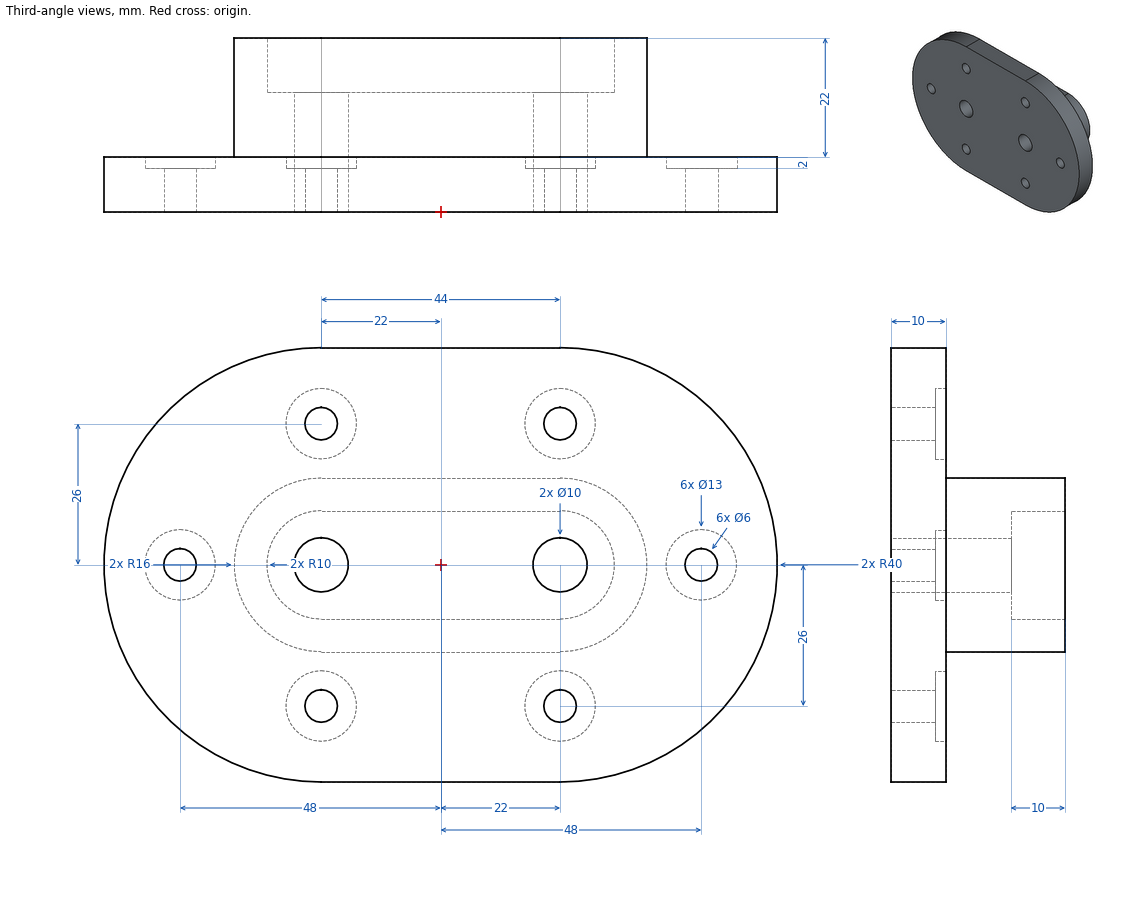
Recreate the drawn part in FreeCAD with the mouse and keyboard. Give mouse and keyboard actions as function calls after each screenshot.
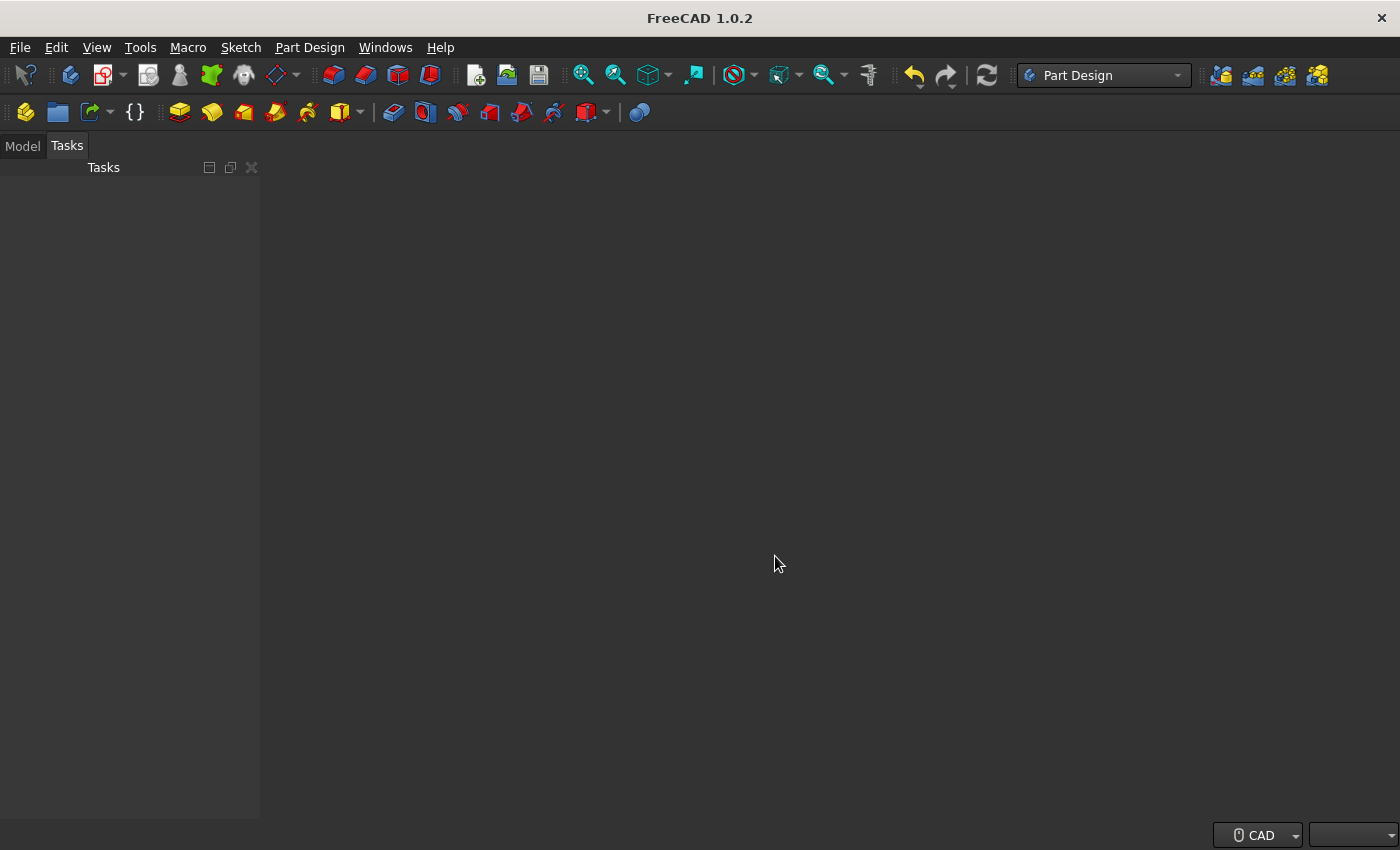
click(476, 76)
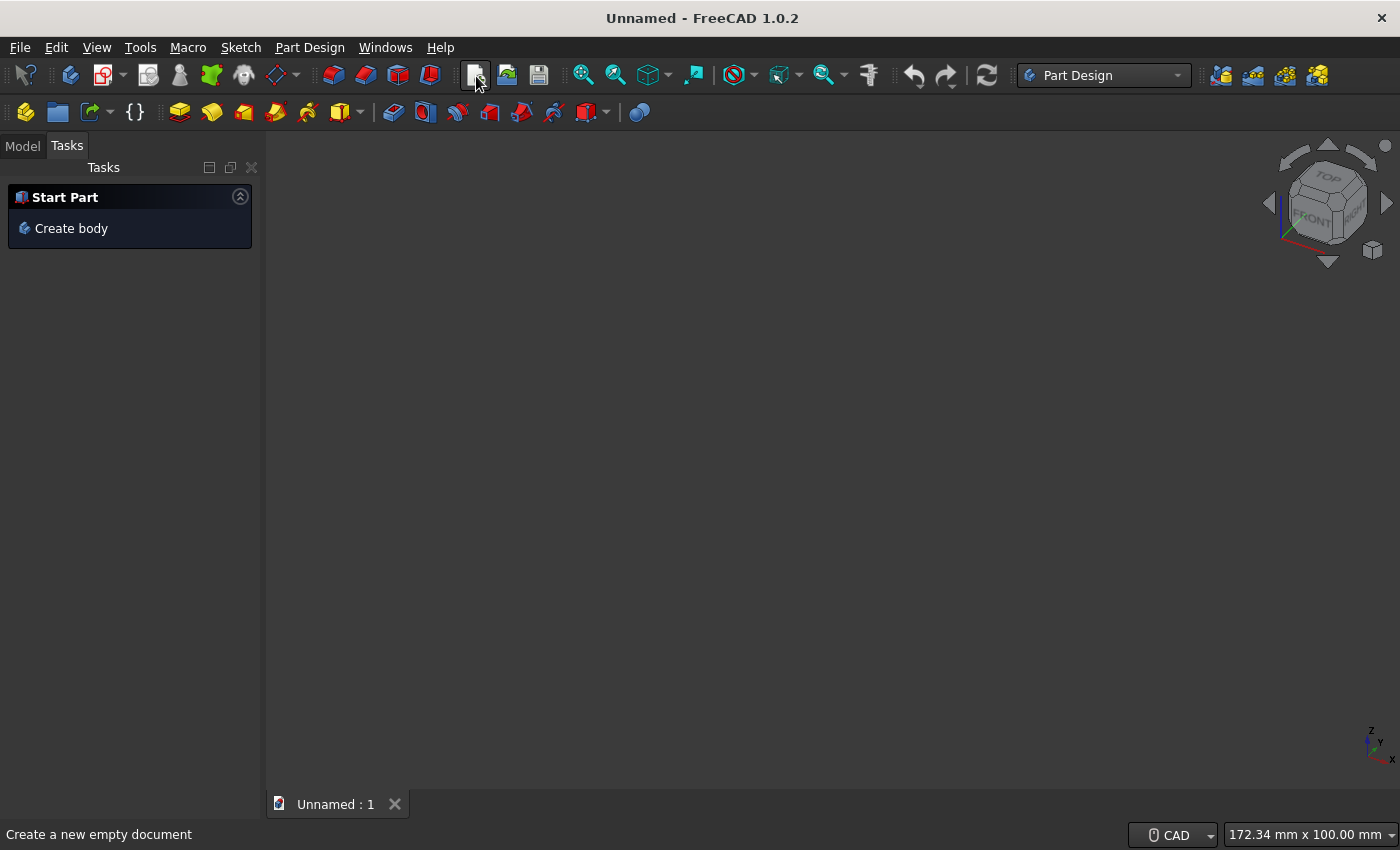
click(104, 76)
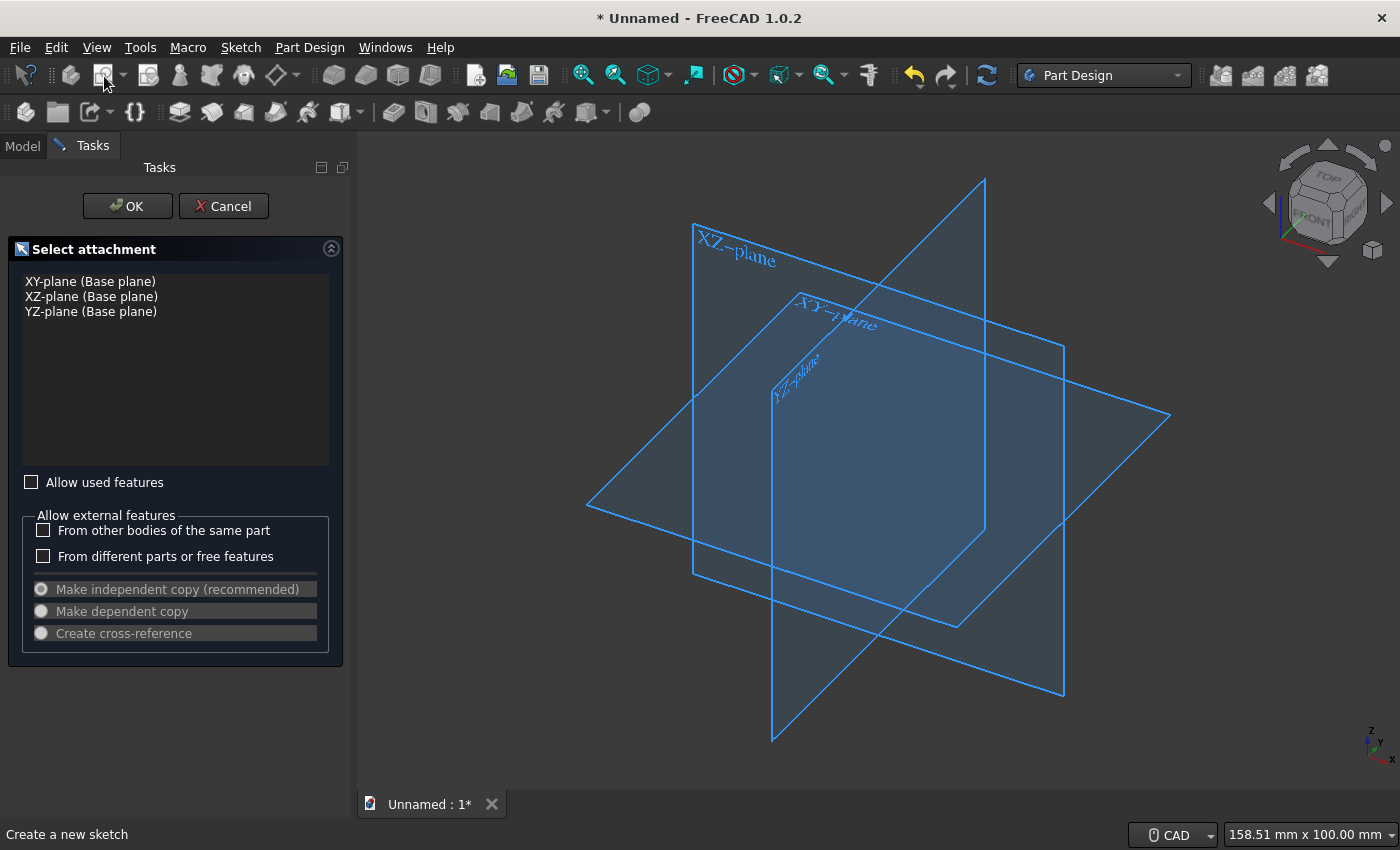
click(82, 296)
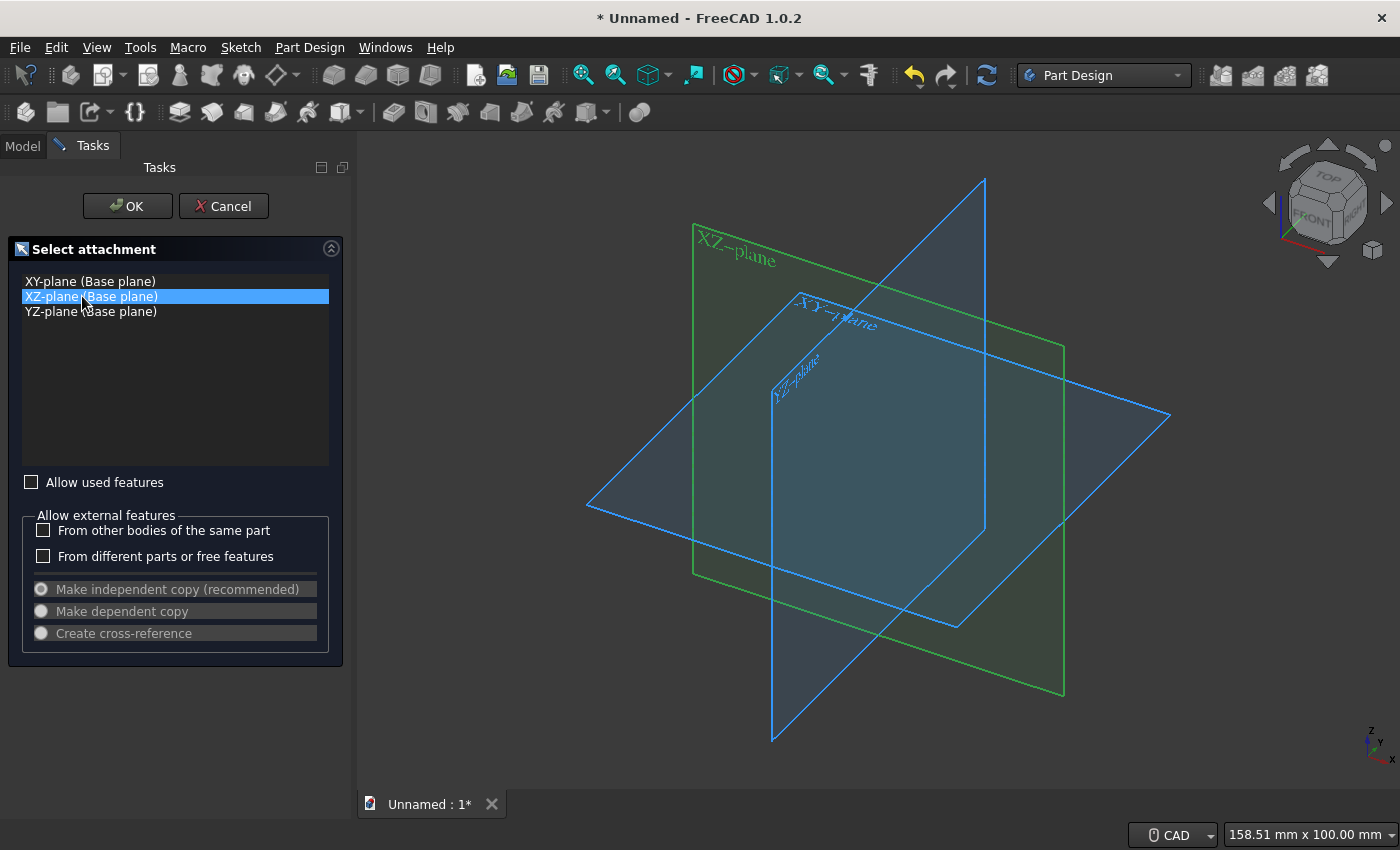
click(128, 206)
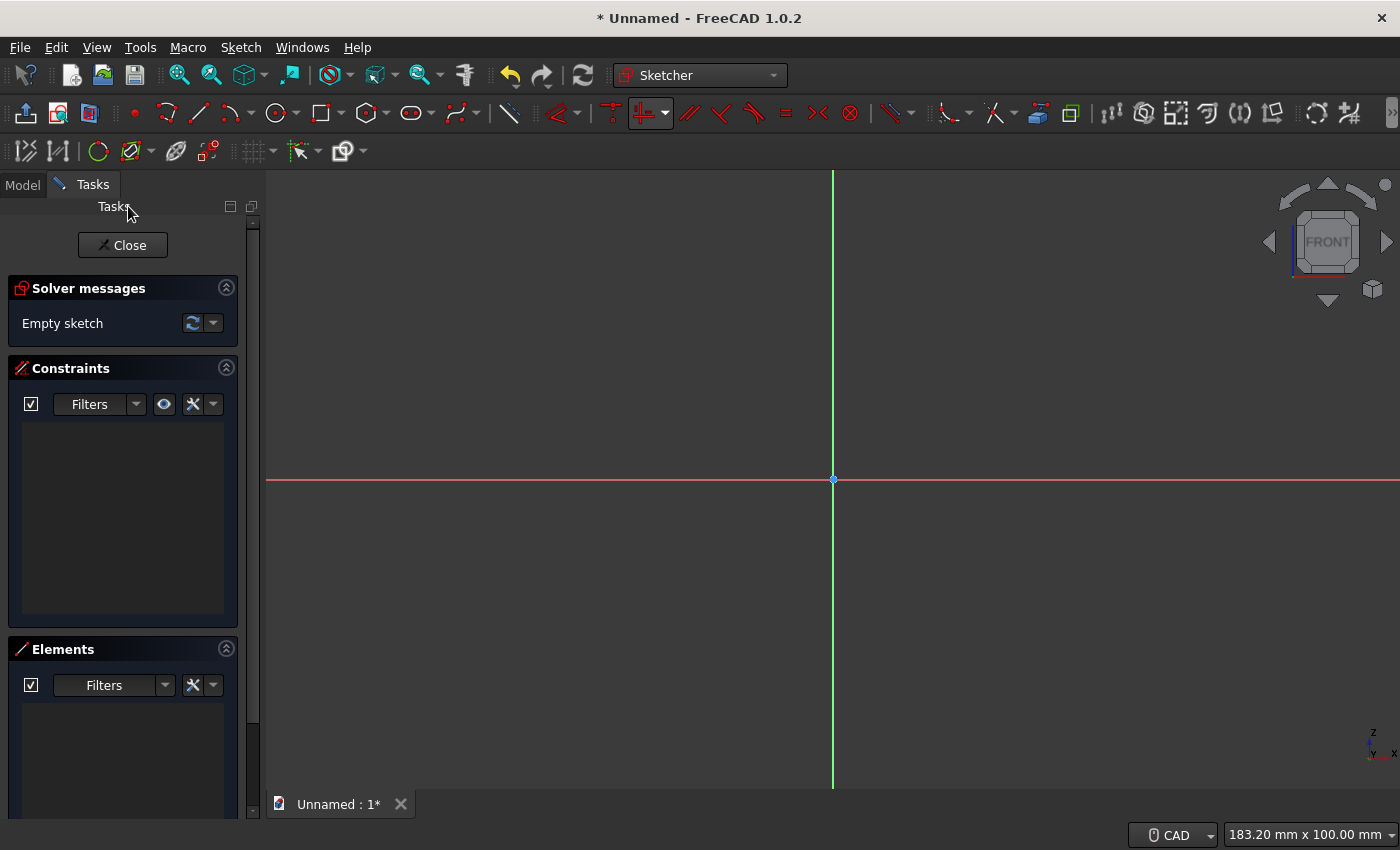
scroll(455, 480, down, 1)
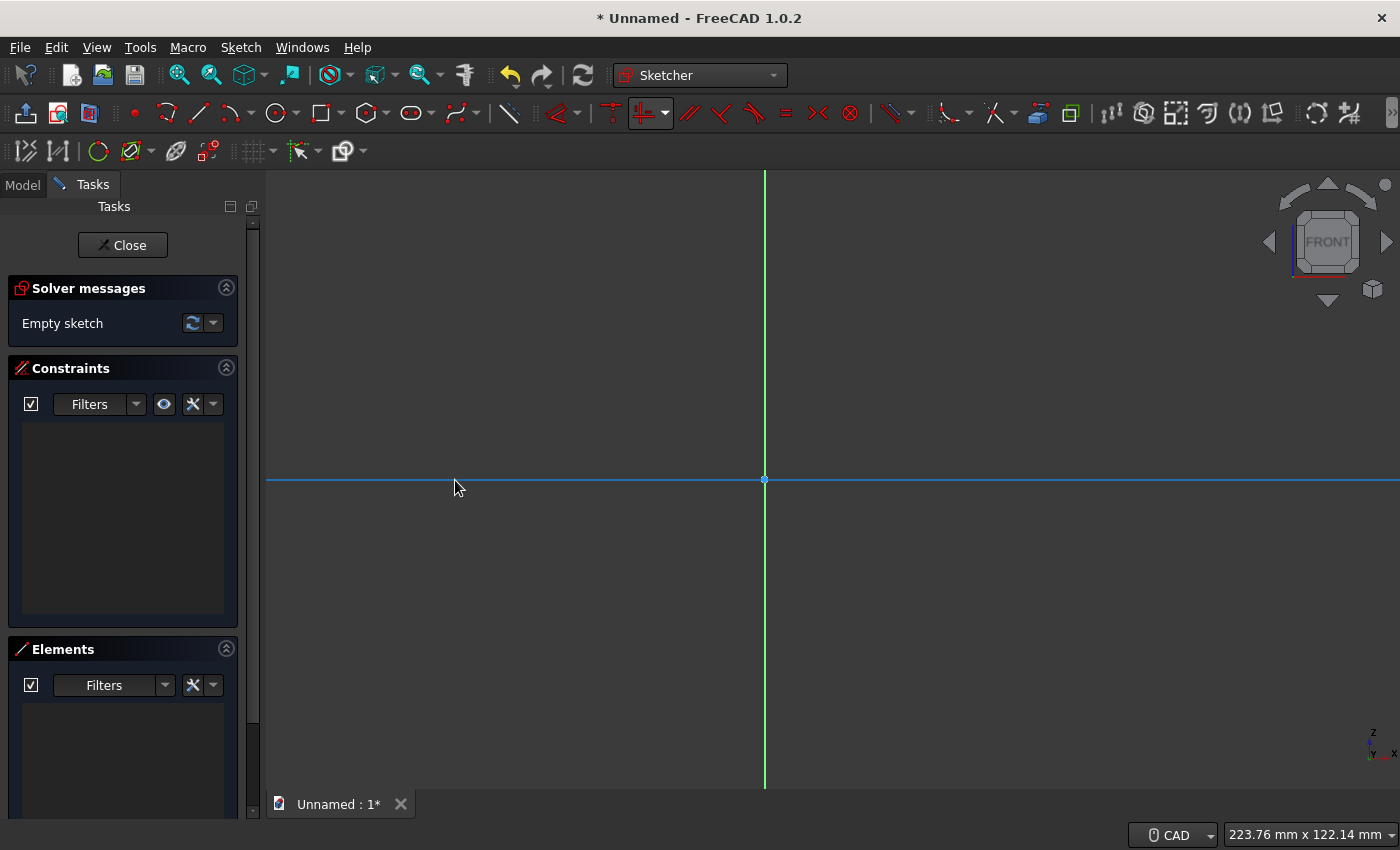
click(412, 114)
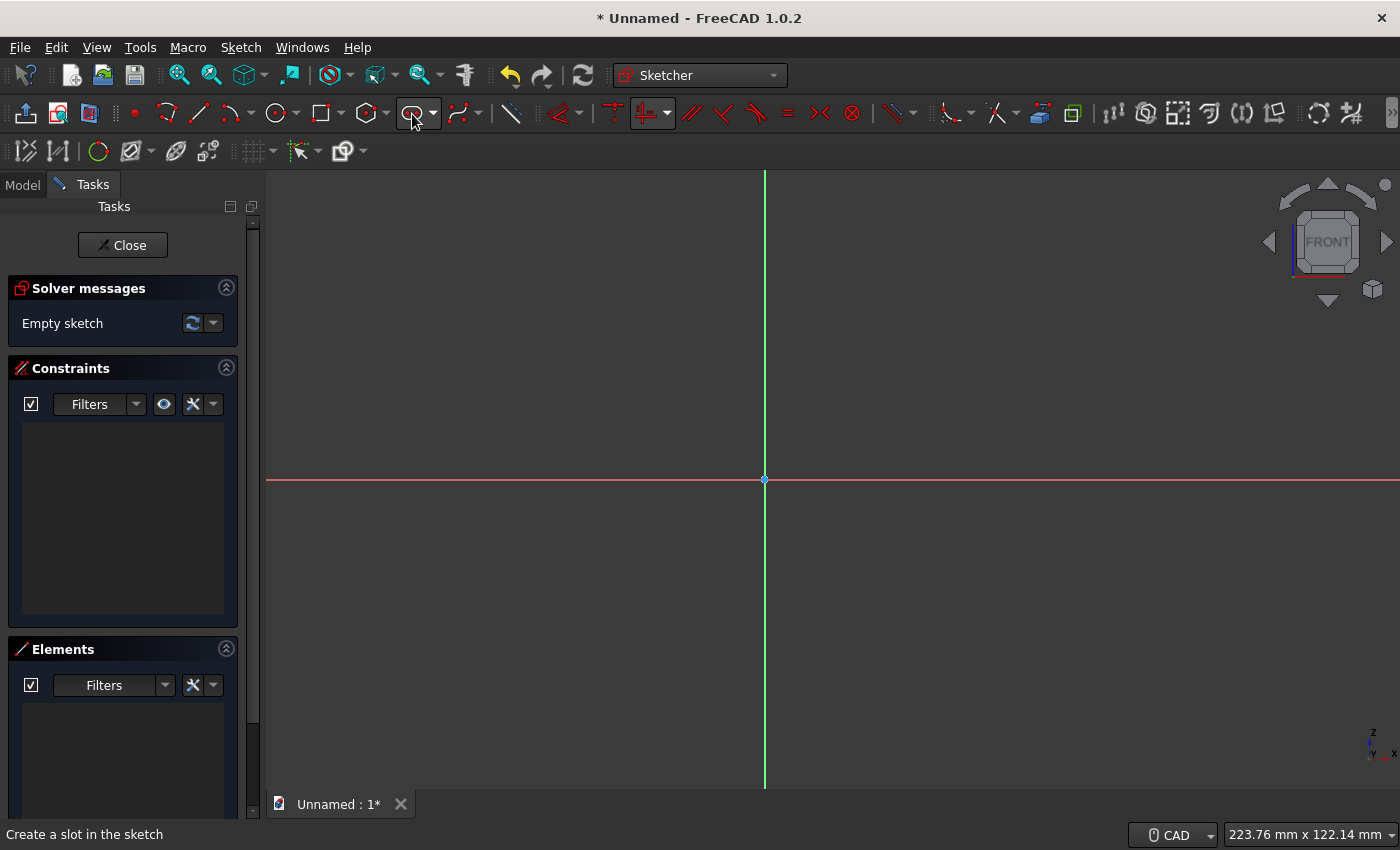
click(653, 480)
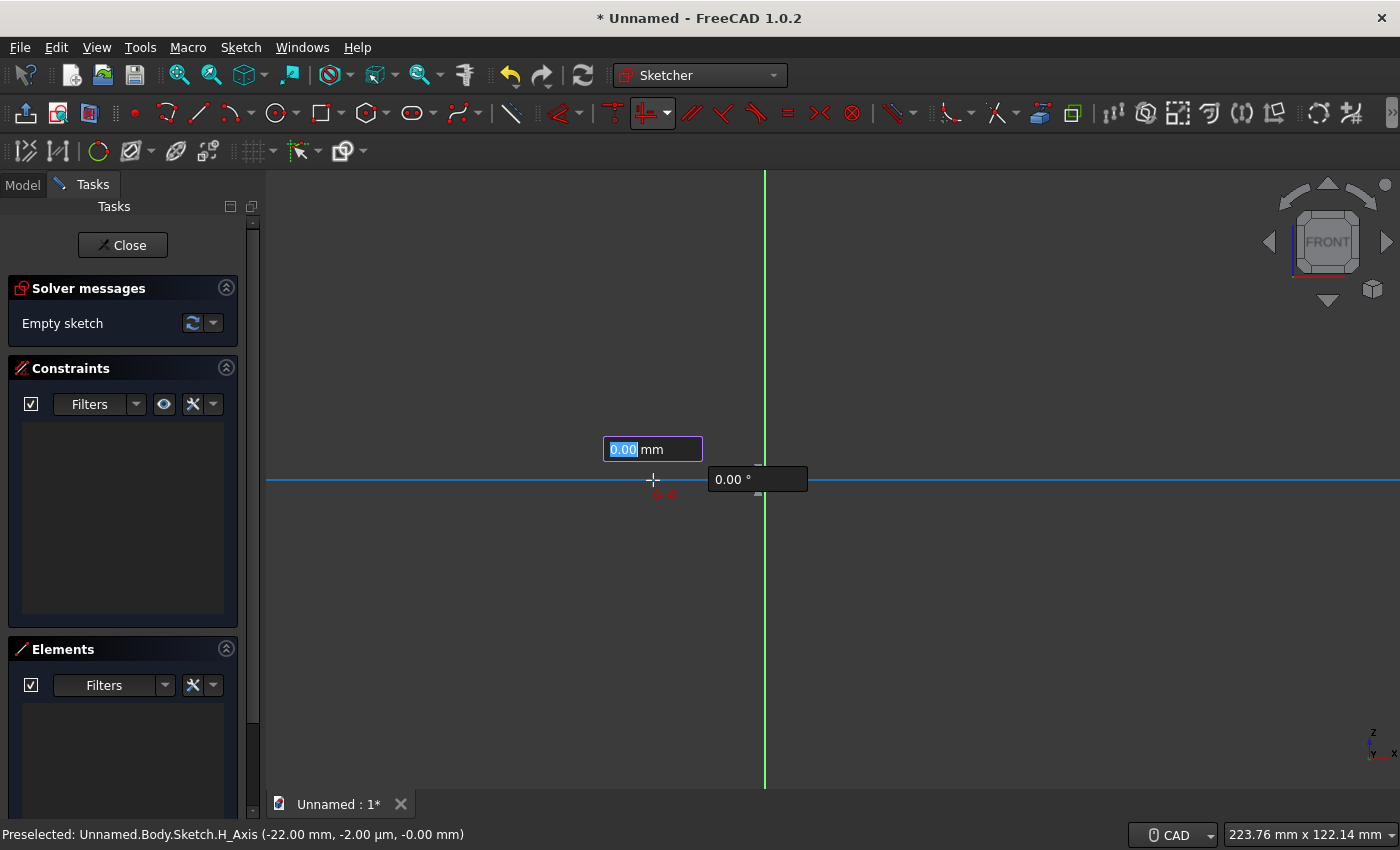
click(876, 471)